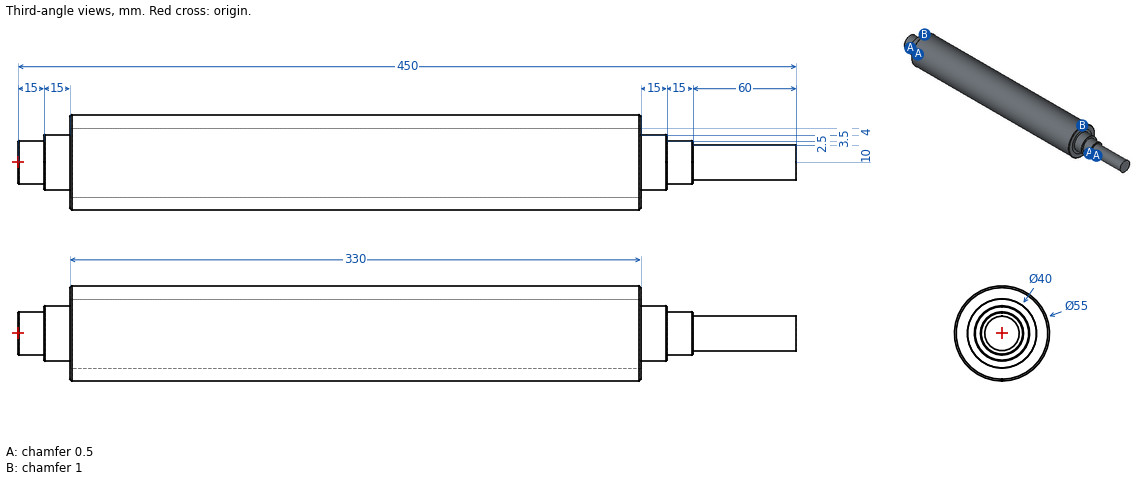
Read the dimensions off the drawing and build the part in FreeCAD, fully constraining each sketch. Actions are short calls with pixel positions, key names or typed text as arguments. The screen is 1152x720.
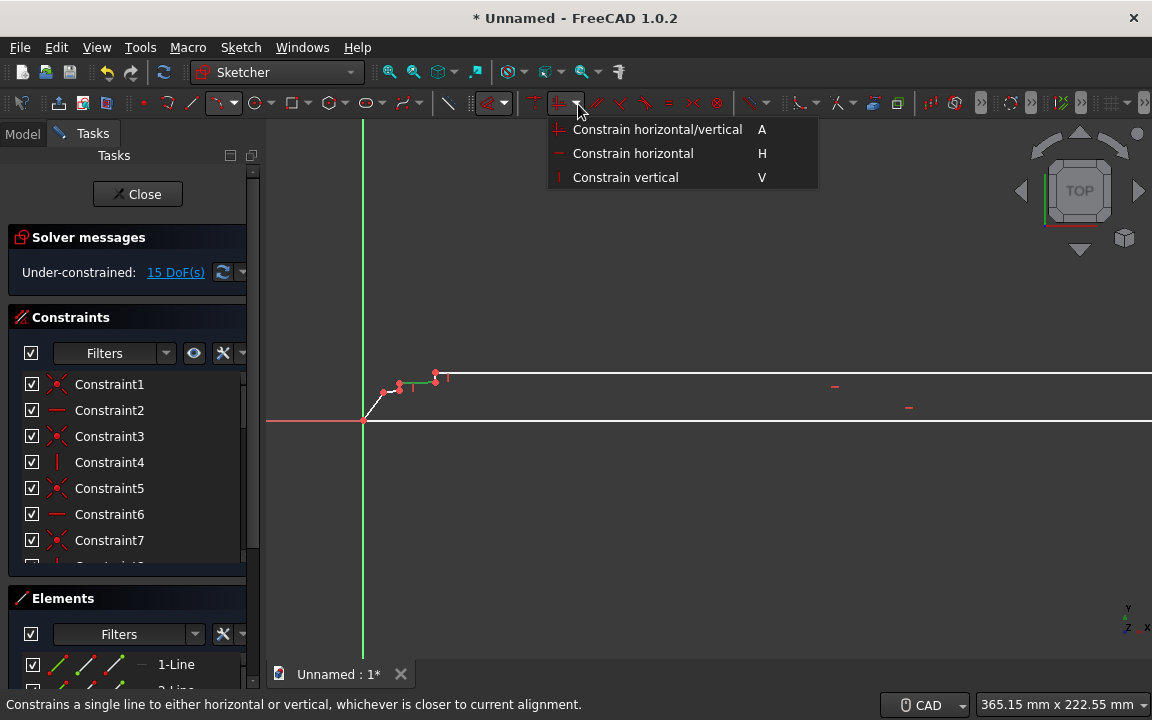
click(683, 153)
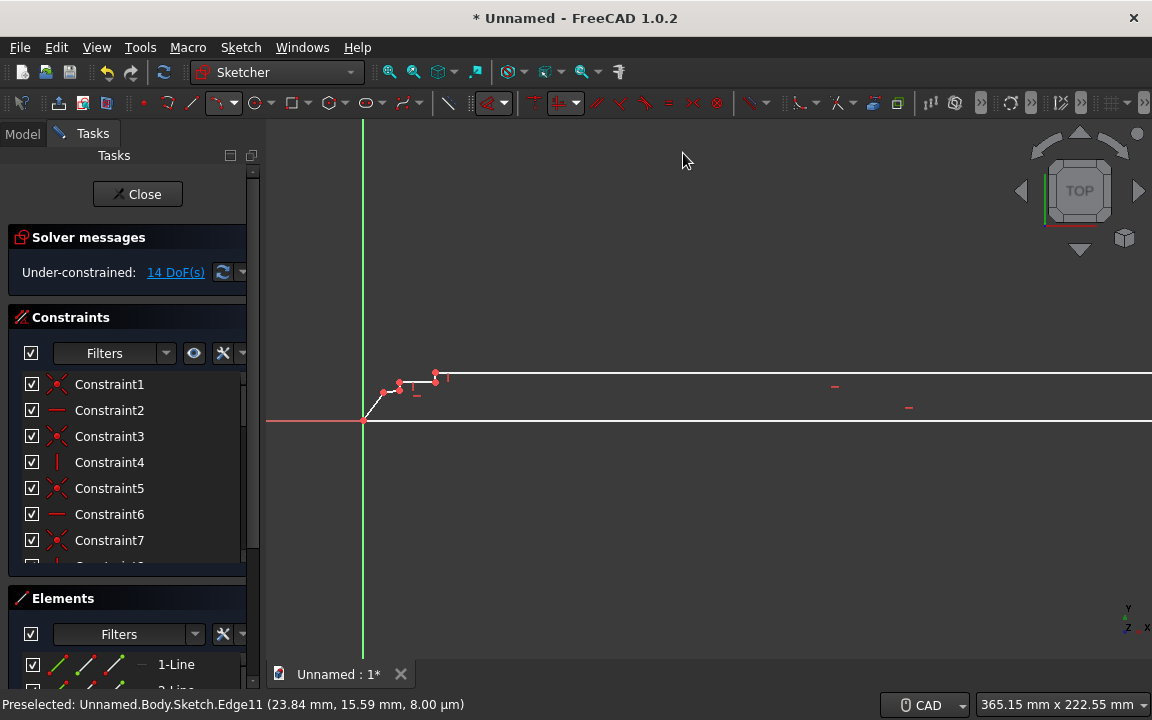
scroll(392, 392, up, 3)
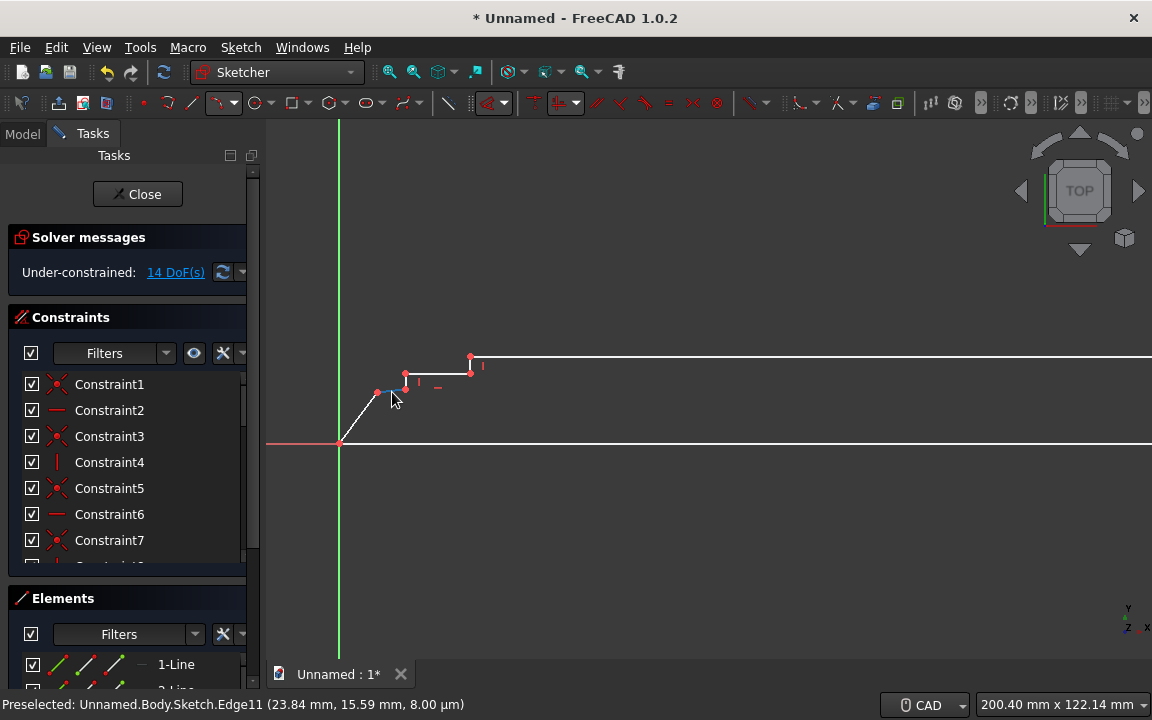
click(391, 391)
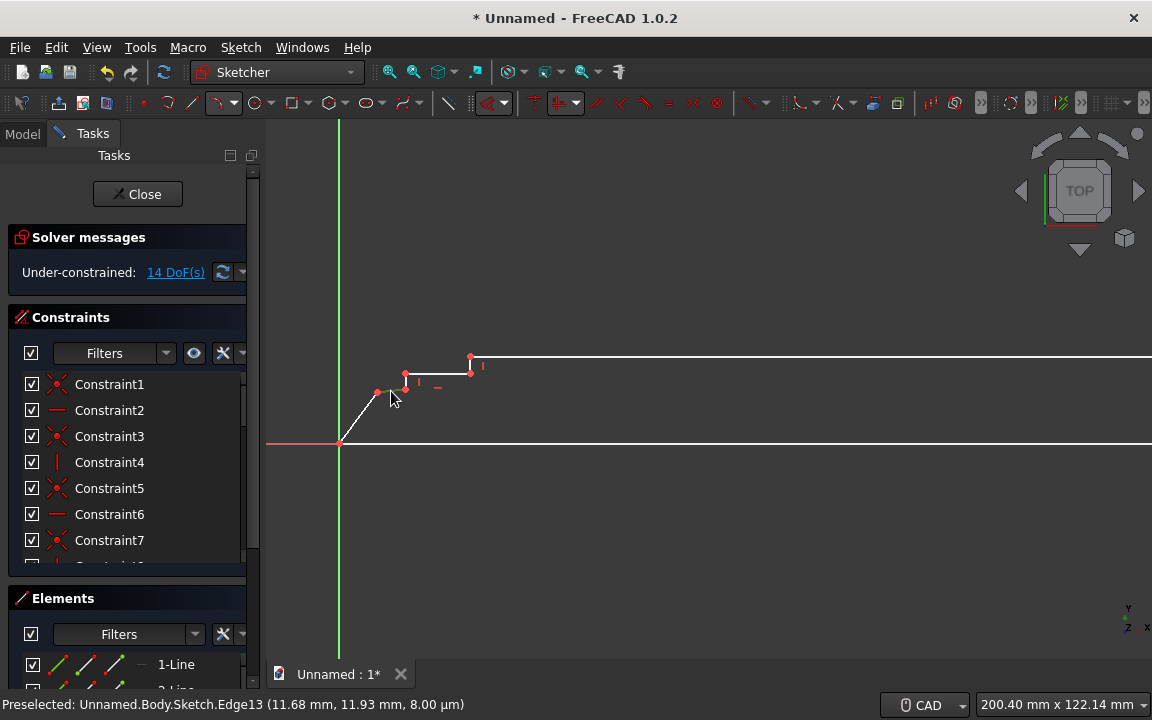
key(h)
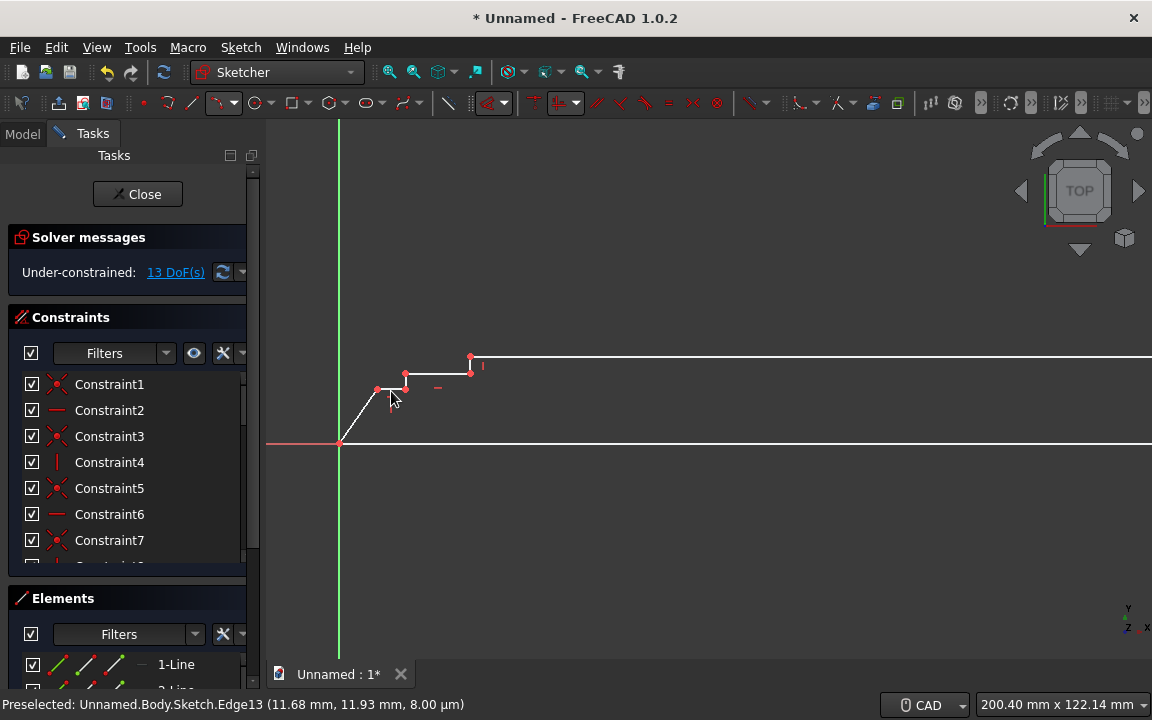
click(366, 406)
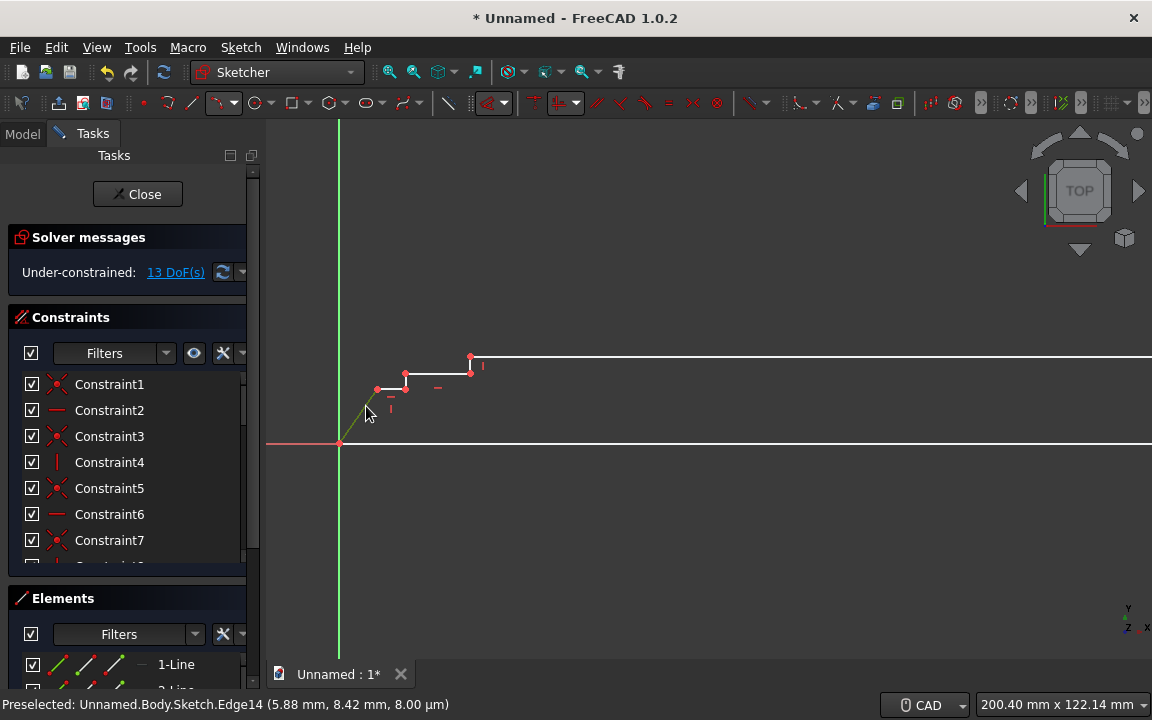
click(578, 104)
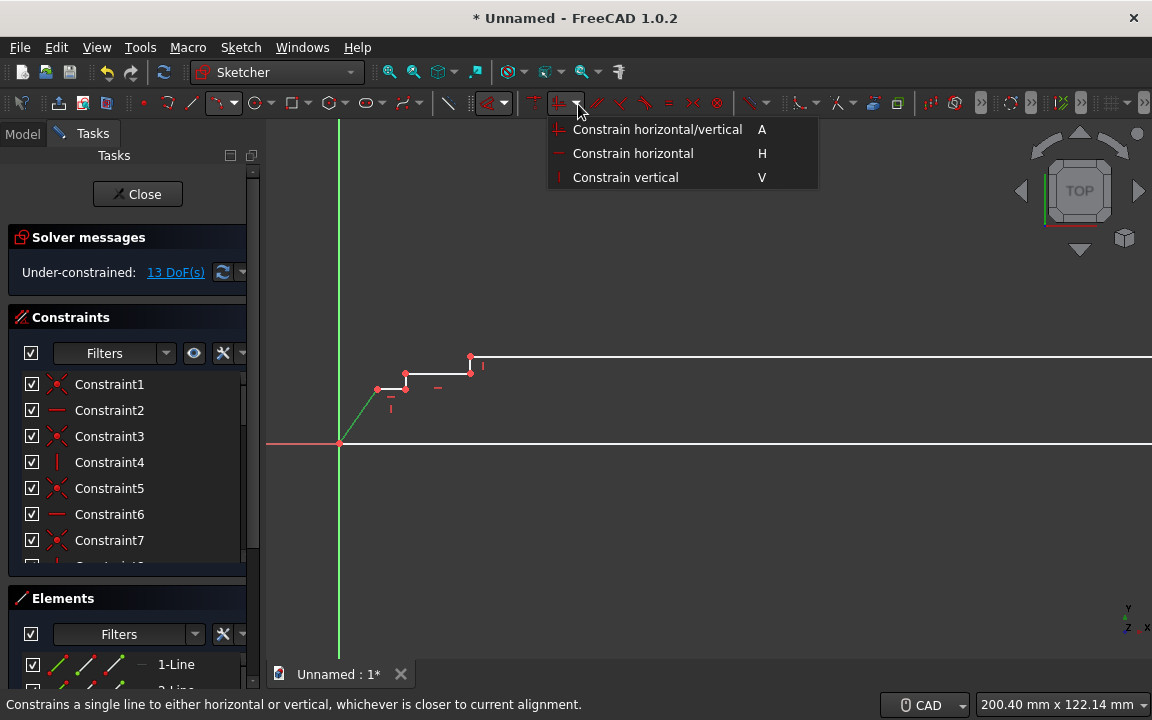
click(683, 177)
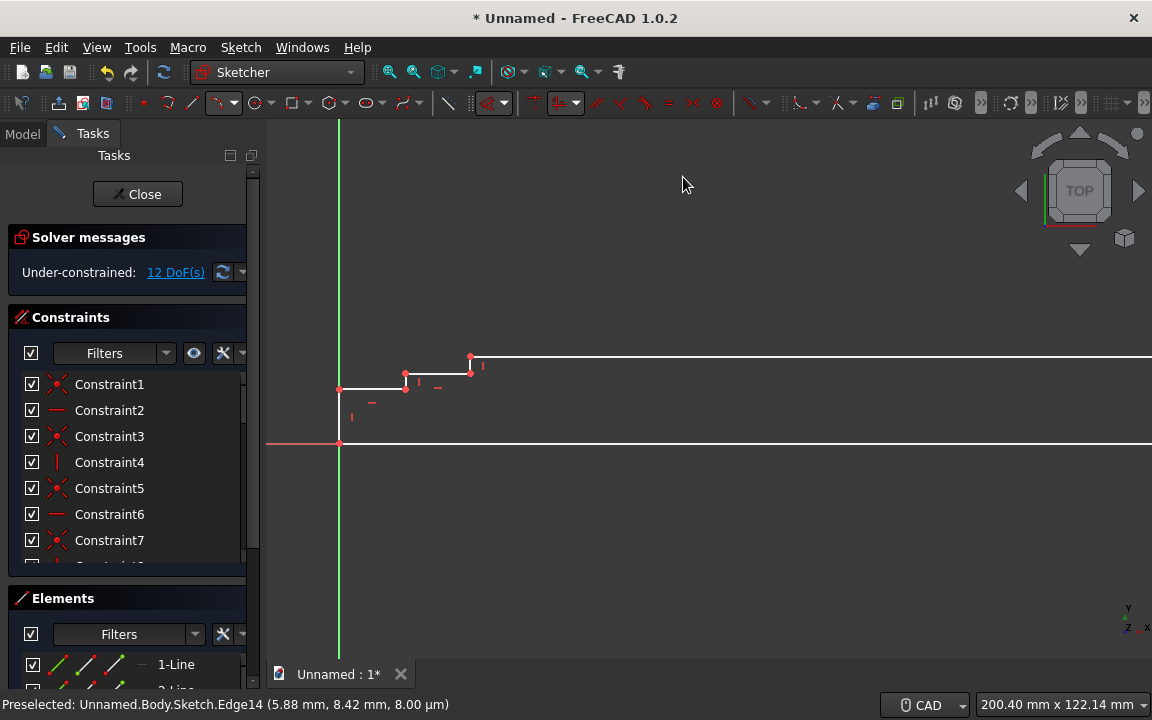
key(d)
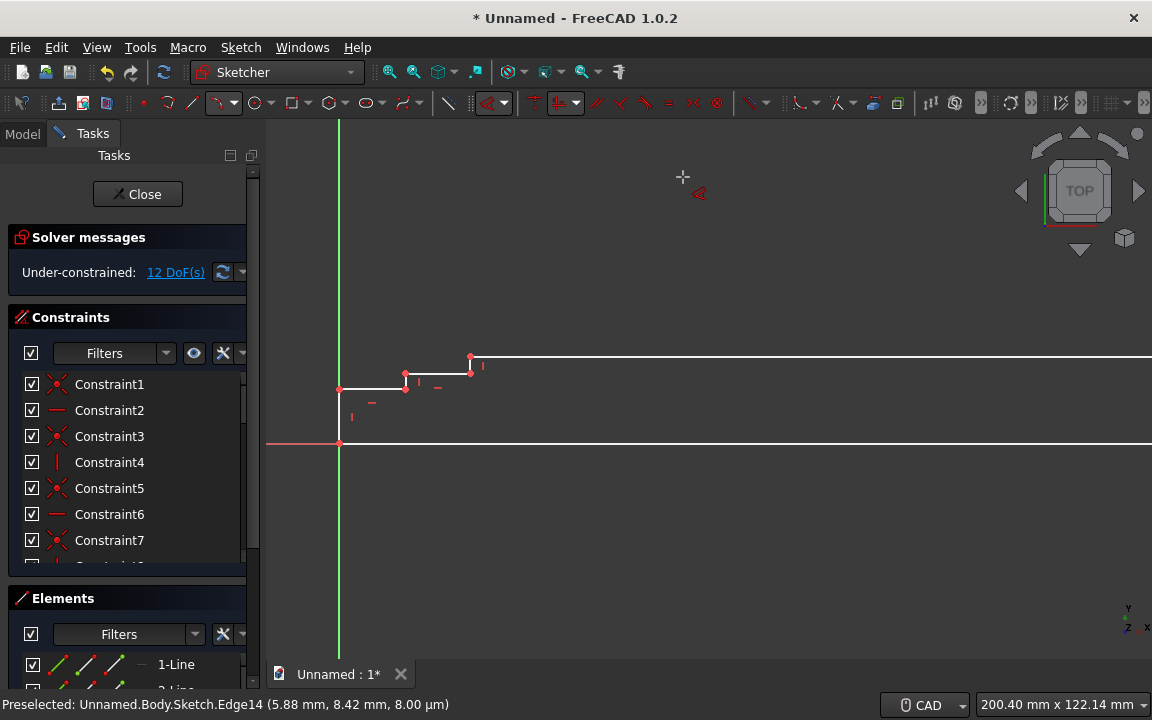
scroll(414, 386, down, 7)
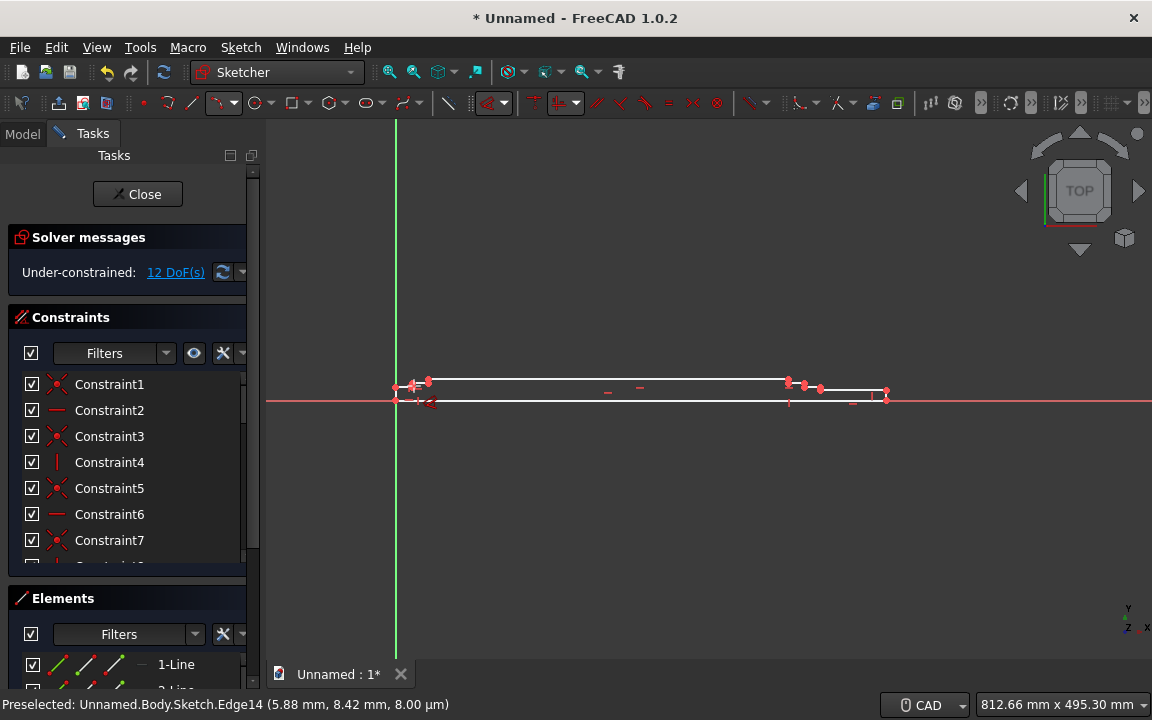
scroll(788, 381, up, 12)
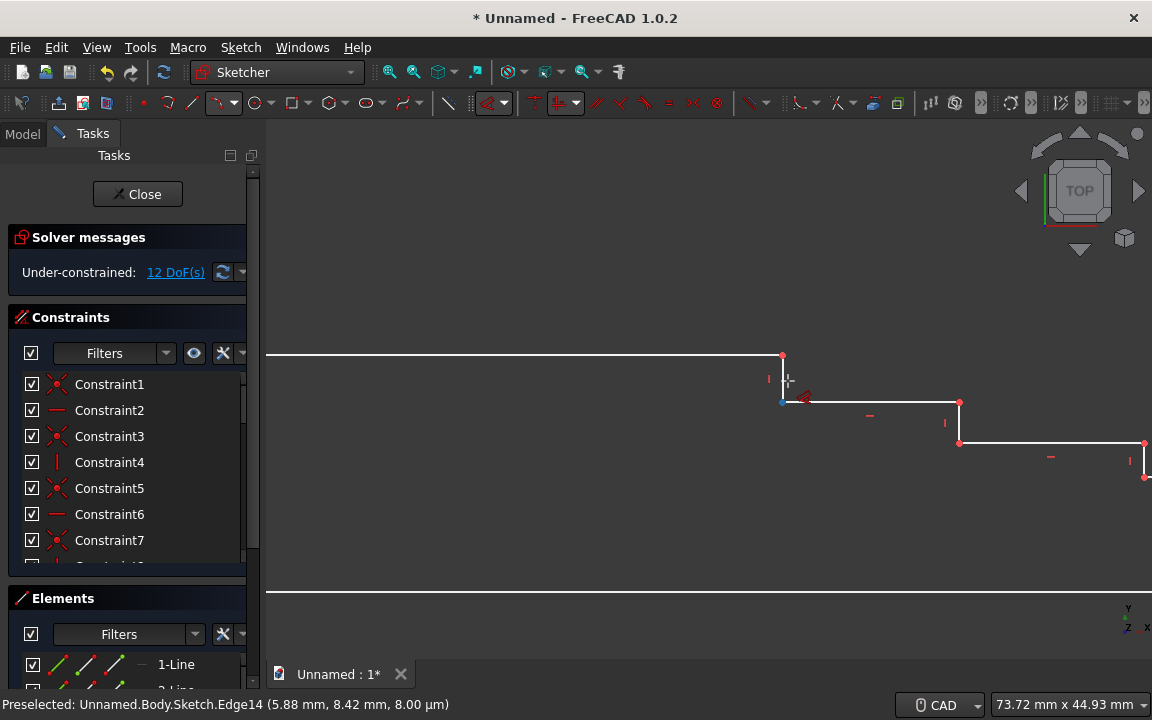
click(783, 379)
click(817, 379)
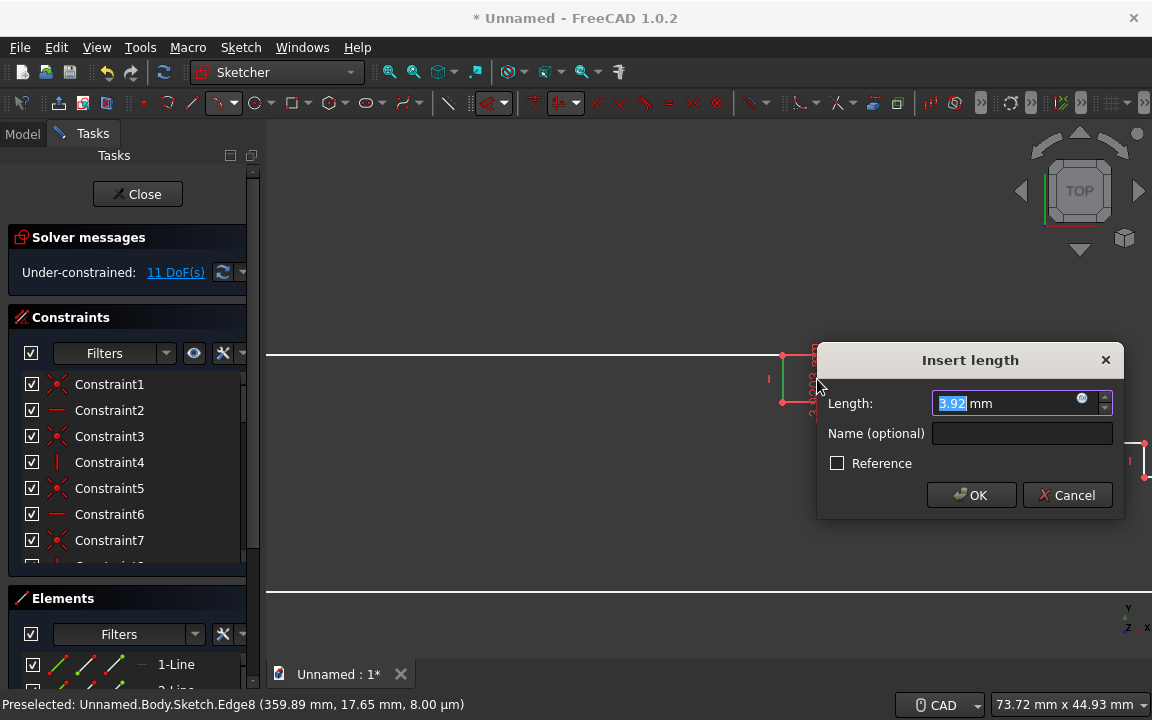
text(4)
key(Return)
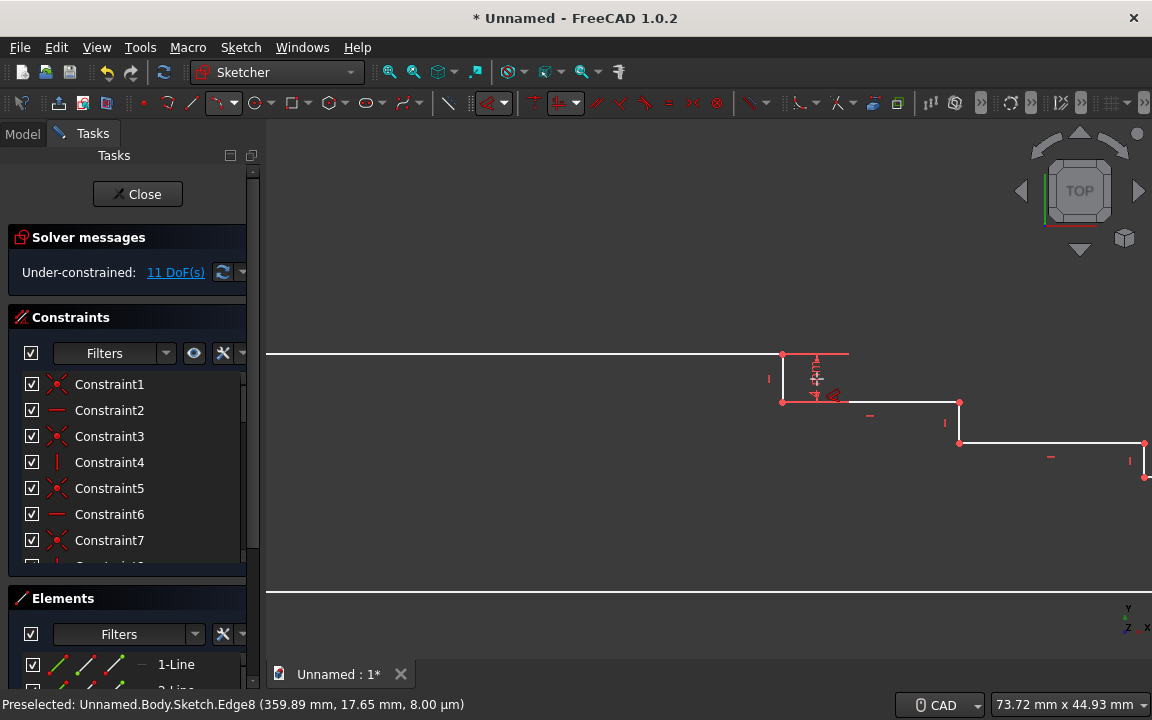
scroll(788, 381, down, 12)